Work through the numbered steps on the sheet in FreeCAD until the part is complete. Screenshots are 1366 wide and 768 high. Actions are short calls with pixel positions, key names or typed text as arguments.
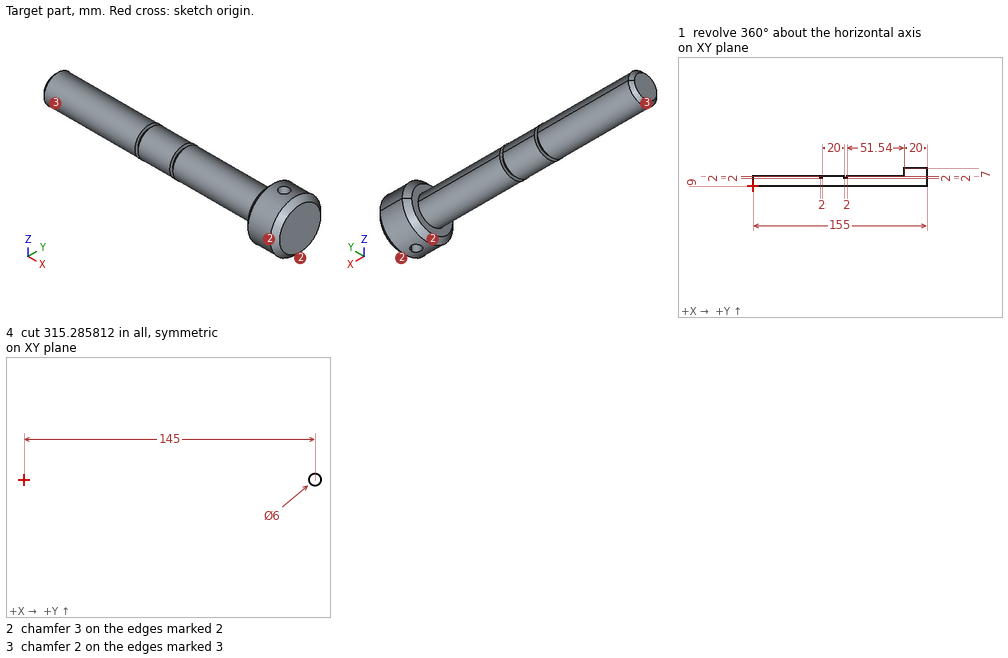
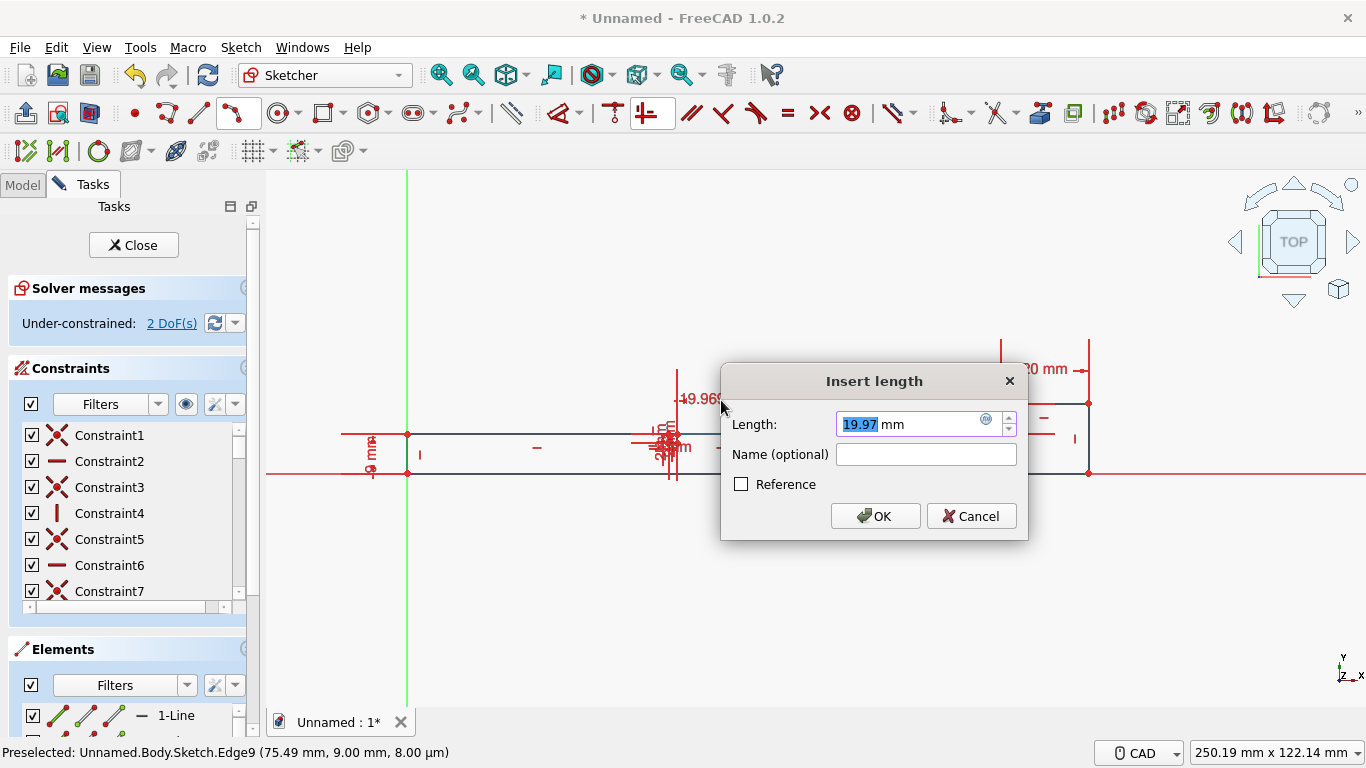
text(20)
key(Return)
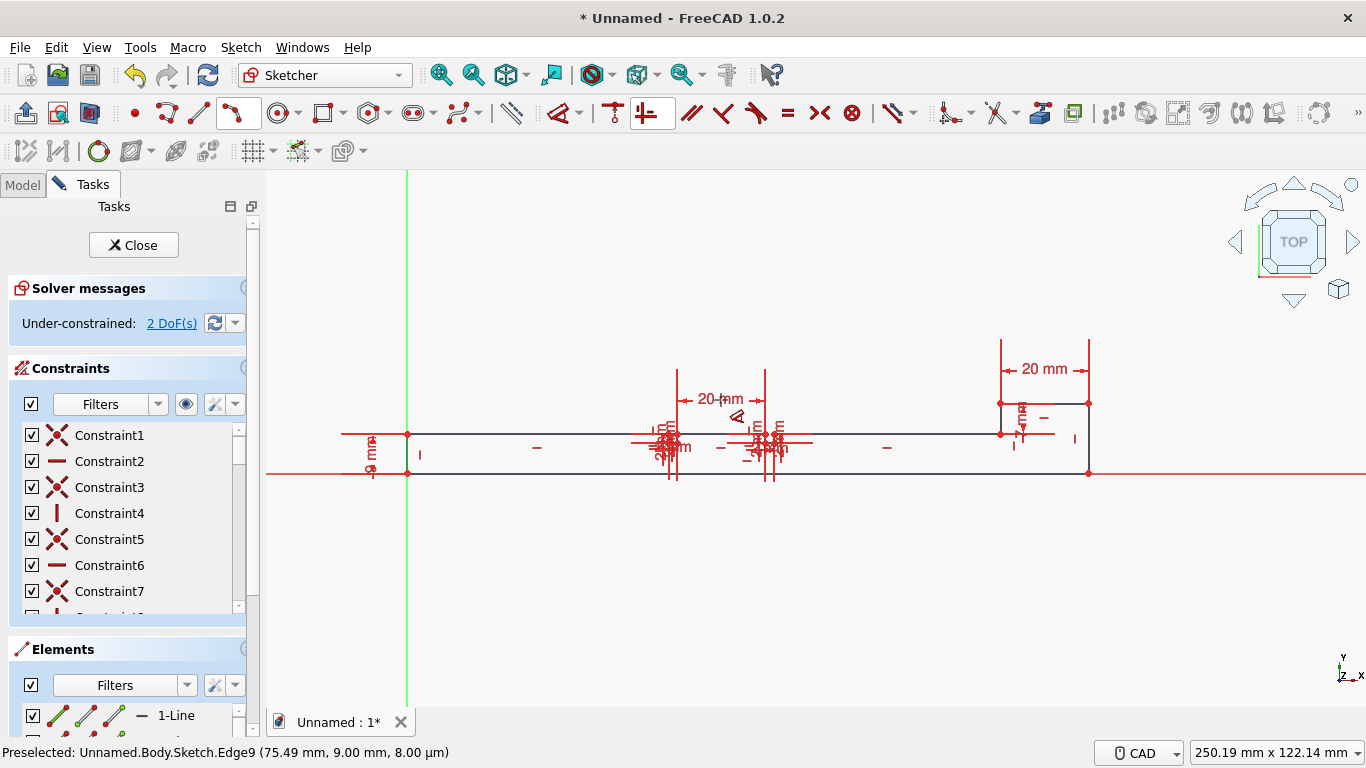
click(612, 474)
click(748, 508)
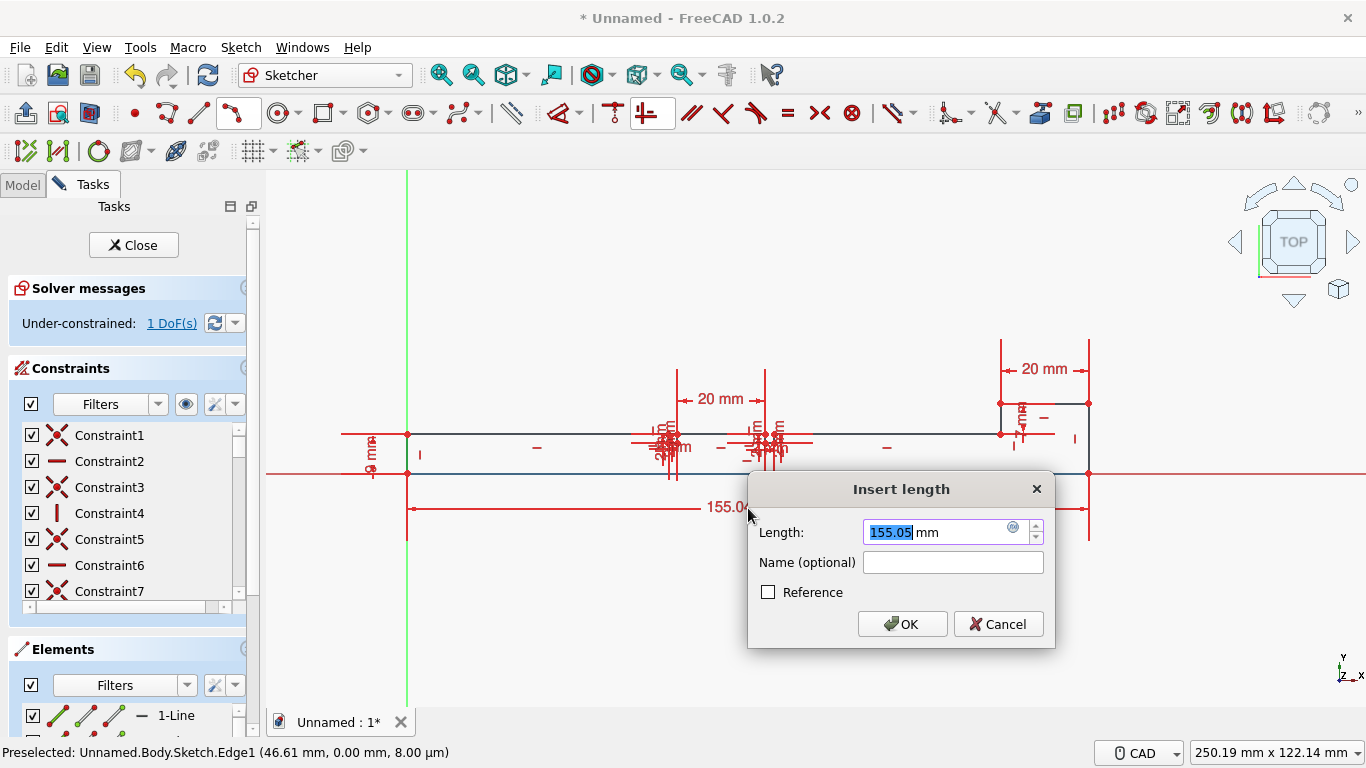
text(155)
key(Return)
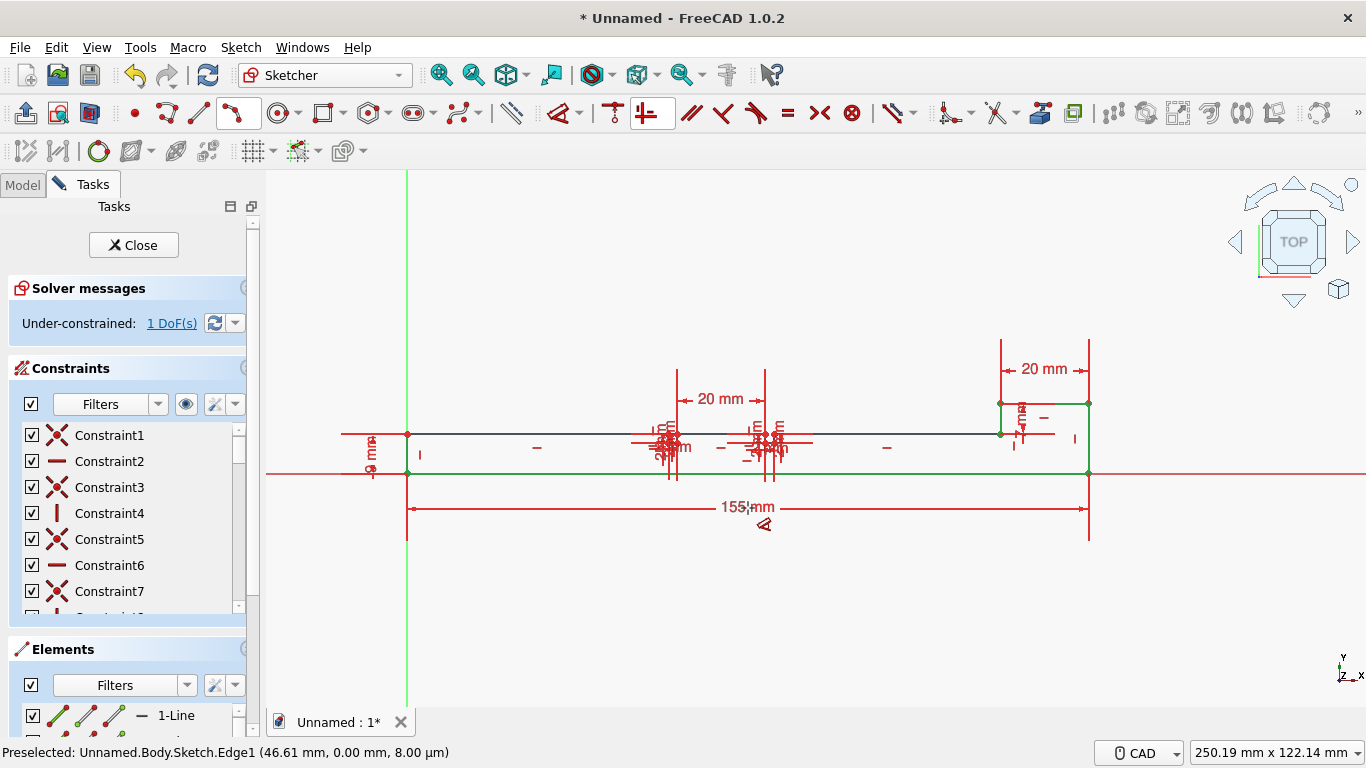
click(933, 434)
click(887, 400)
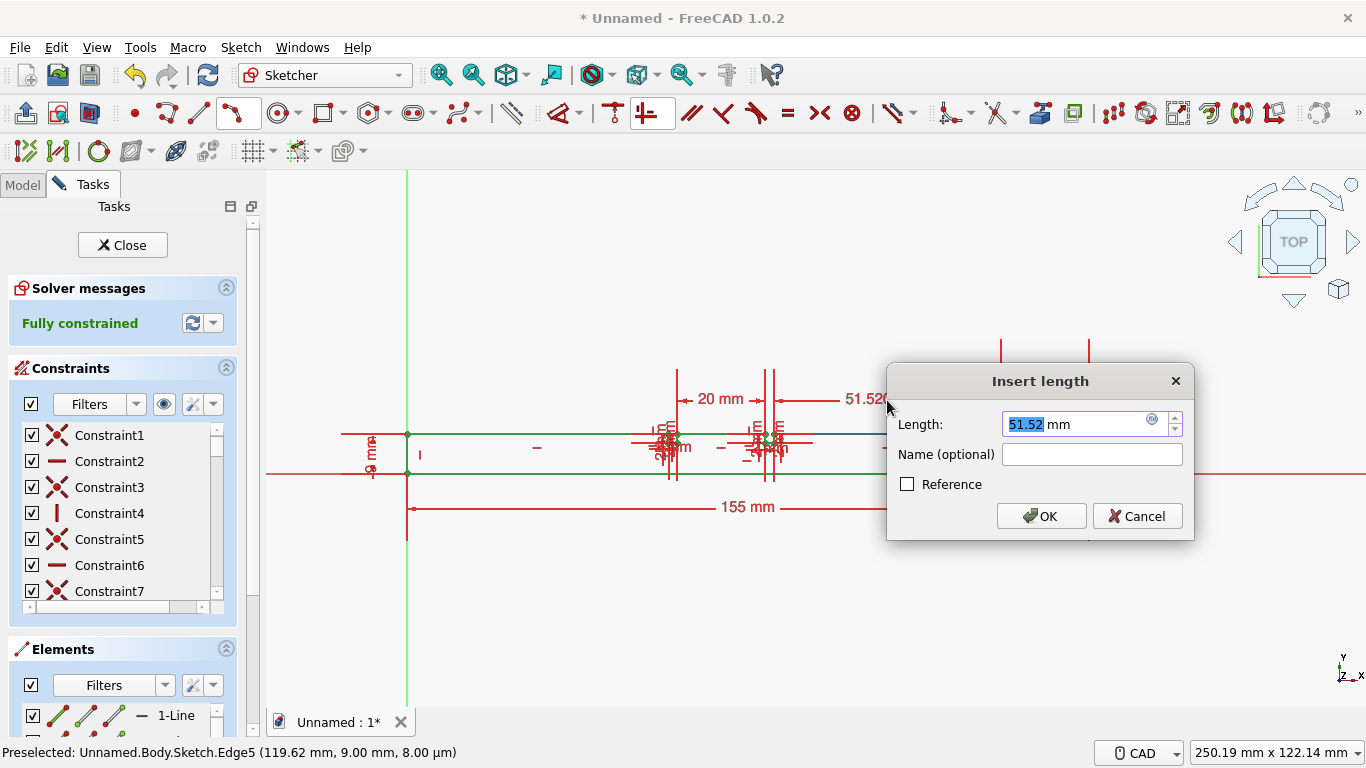
text(51.54)
key(Return)
key(Escape)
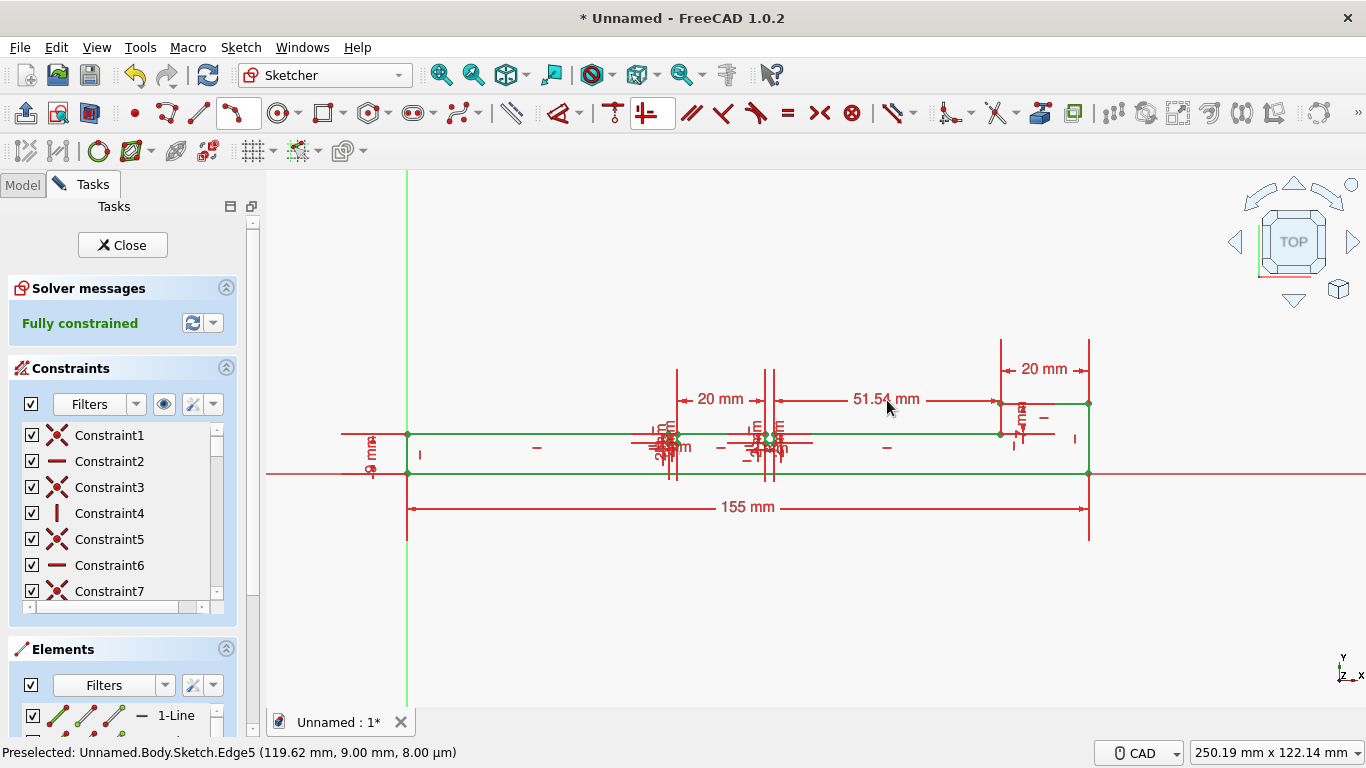
click(123, 245)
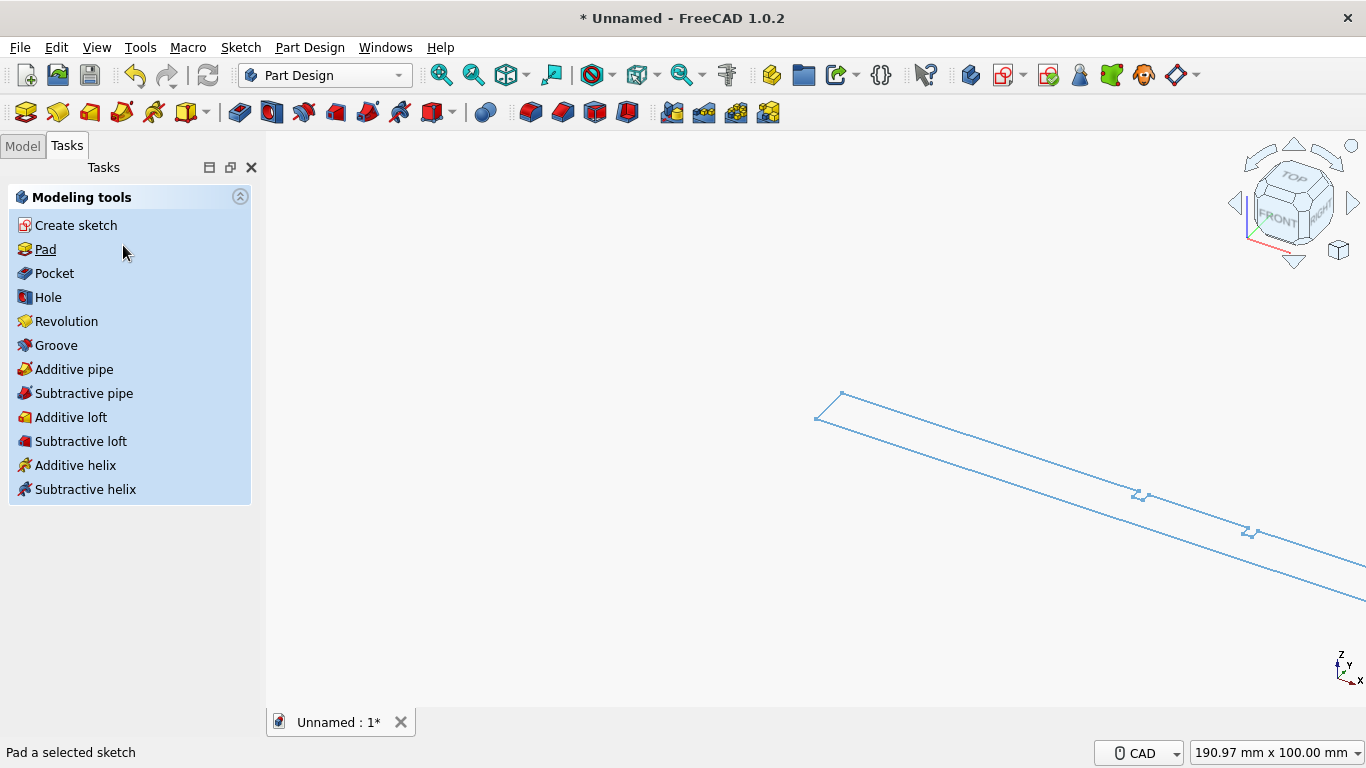
click(58, 112)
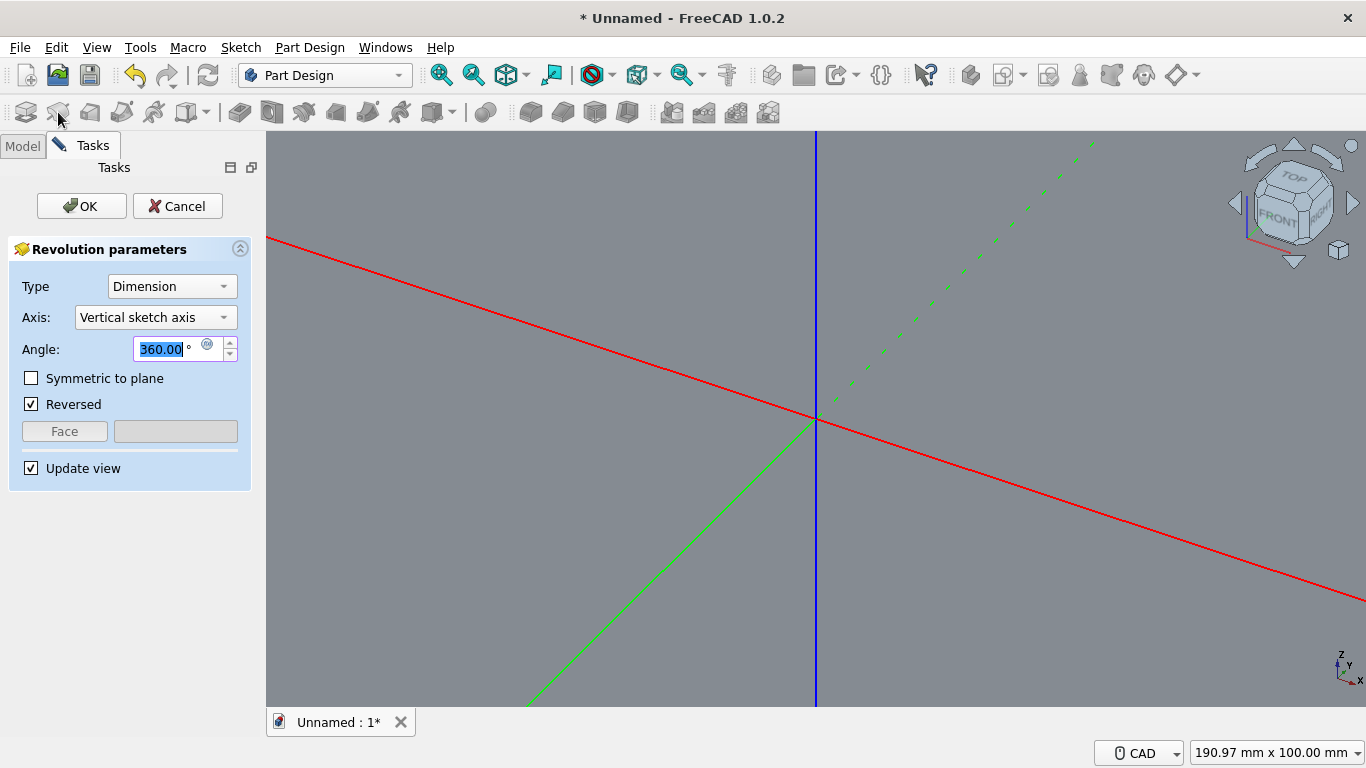
click(156, 318)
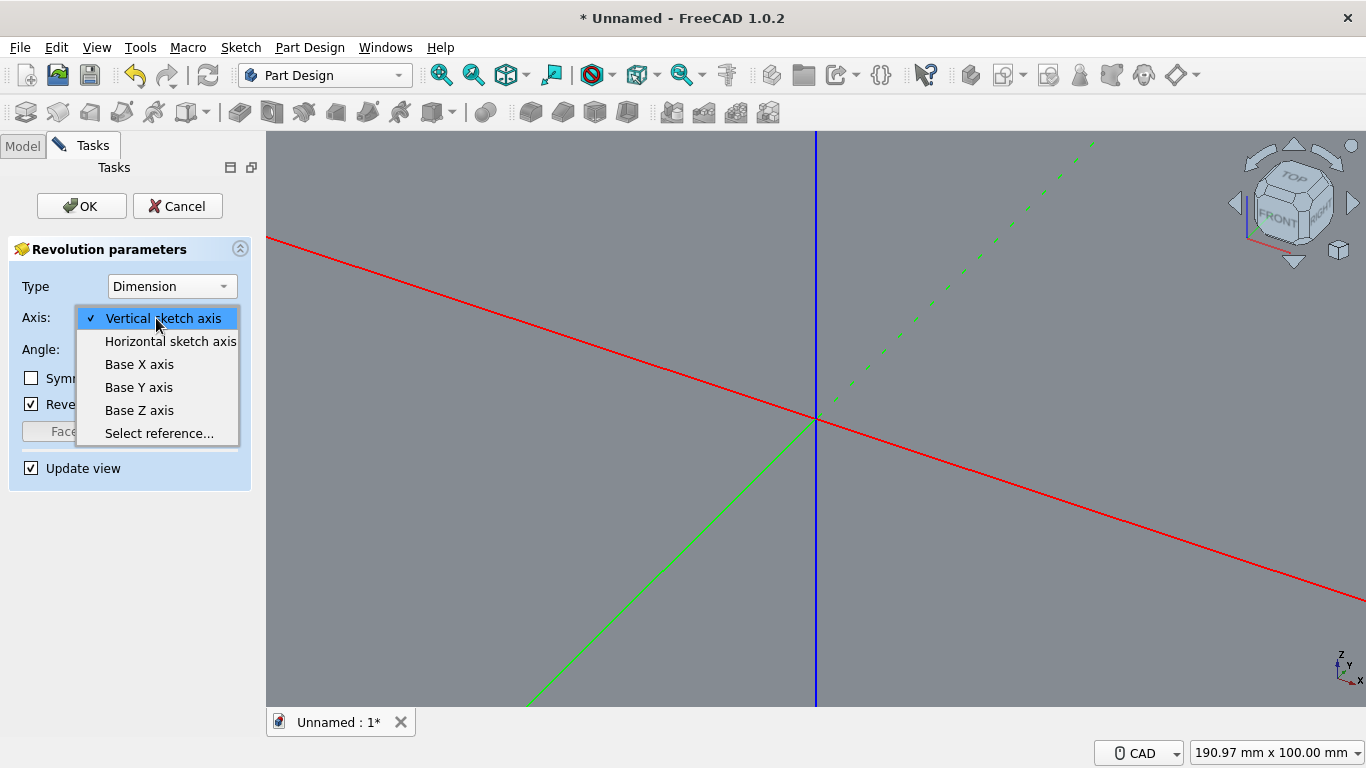
click(156, 342)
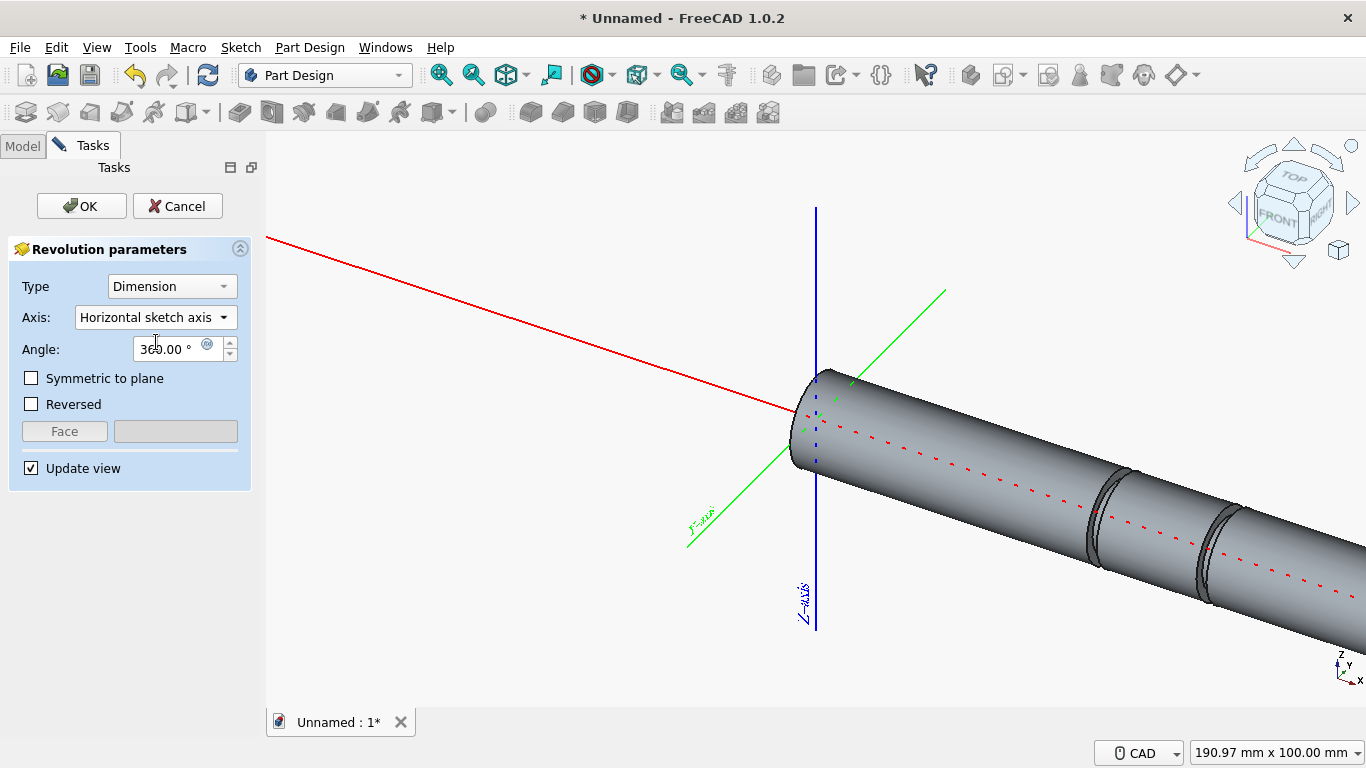
click(82, 206)